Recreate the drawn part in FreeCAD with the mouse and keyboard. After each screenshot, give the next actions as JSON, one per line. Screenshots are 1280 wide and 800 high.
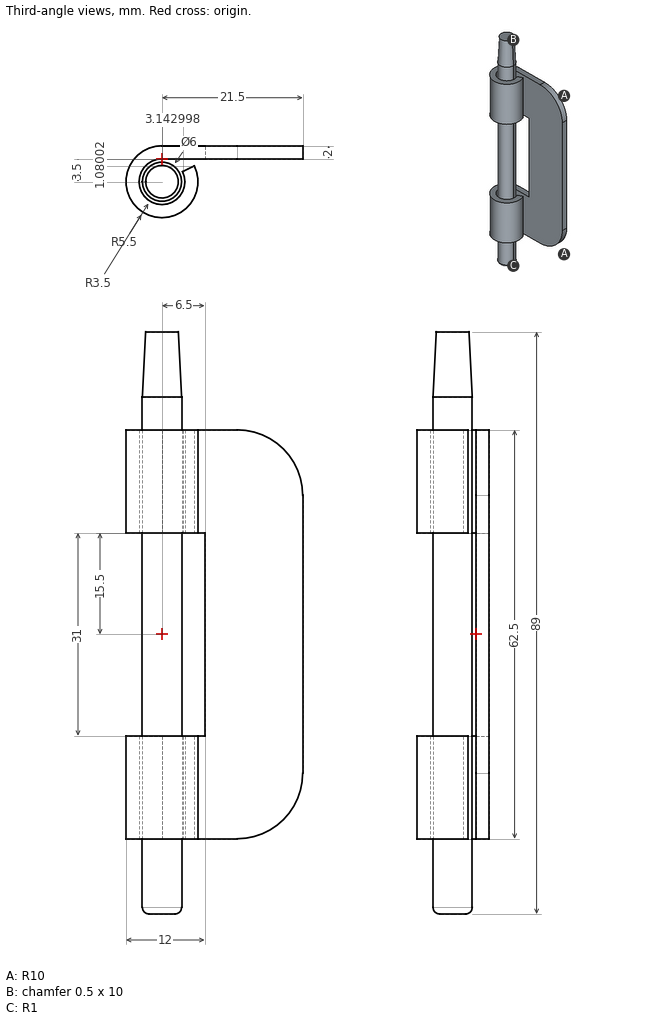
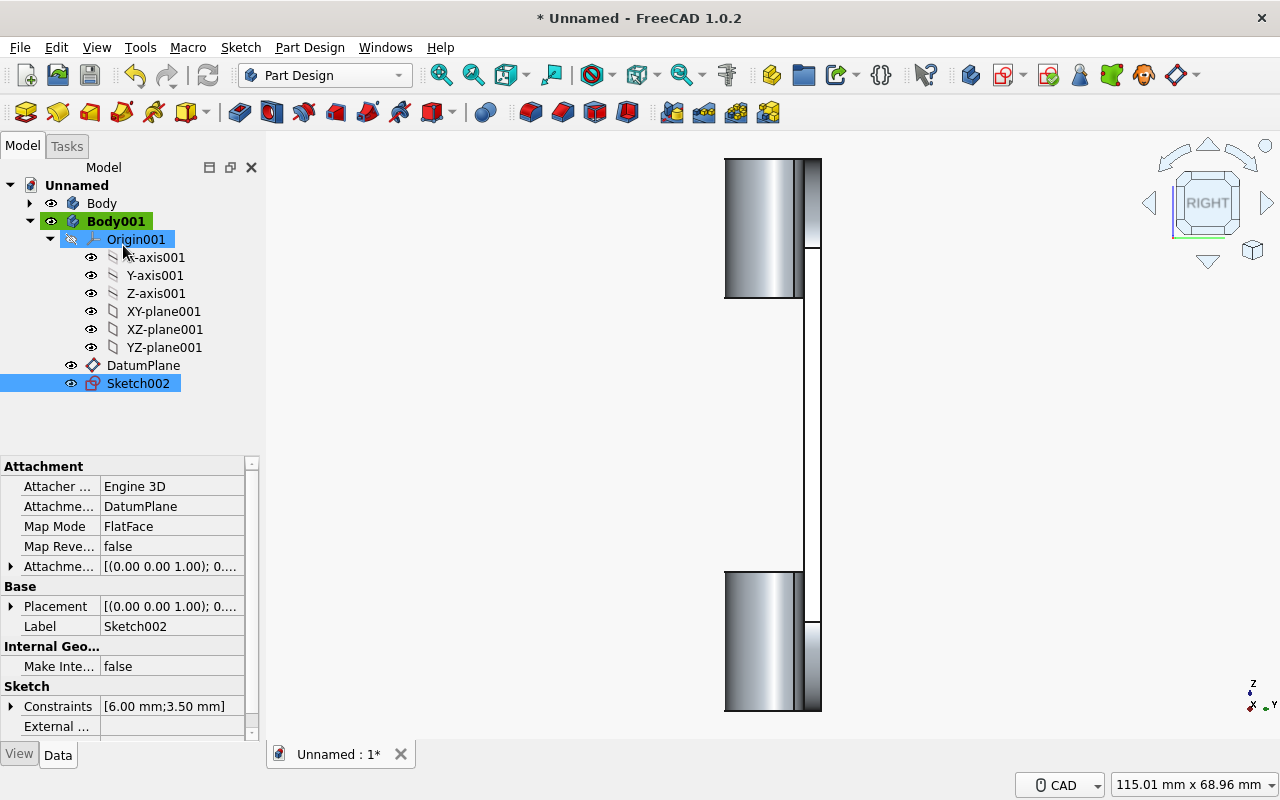
{"action": "left_click", "coordinate": [26, 112]}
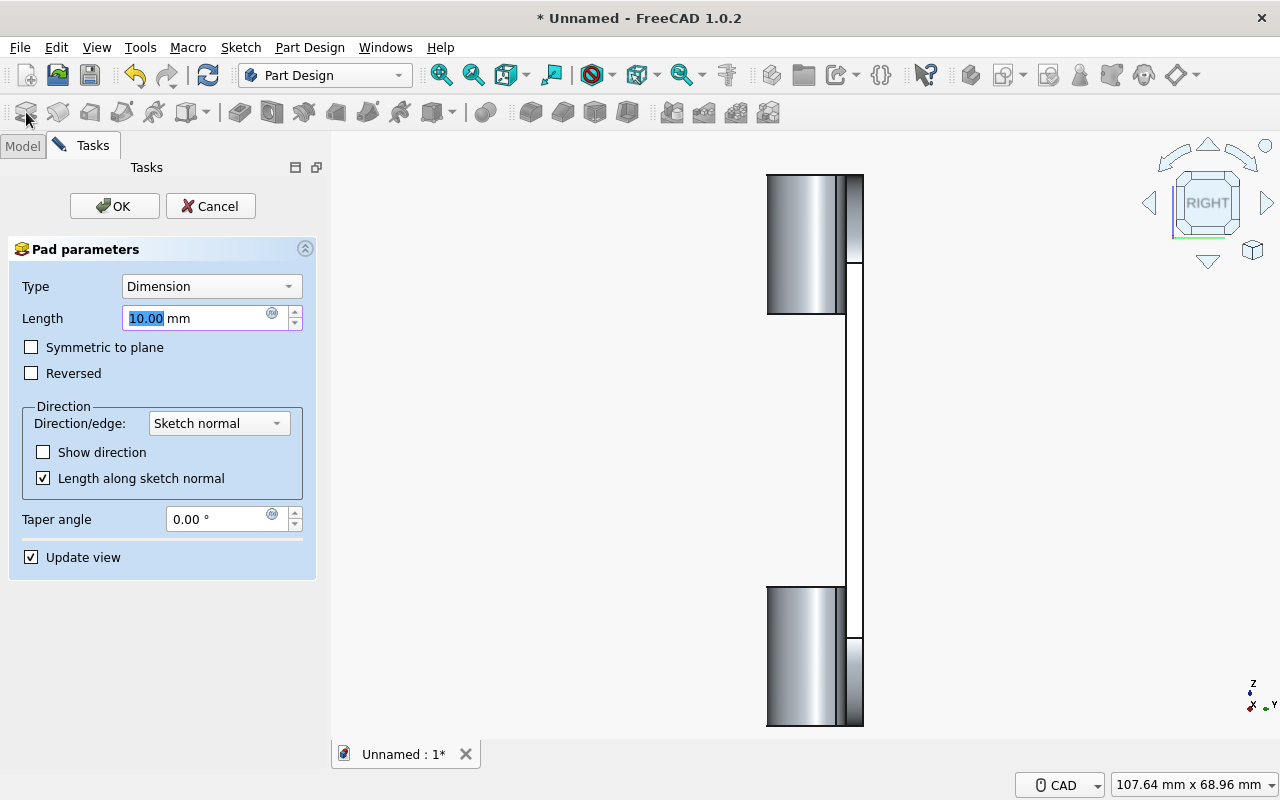
{"action": "type", "text": "89"}
{"action": "key", "text": "Tab"}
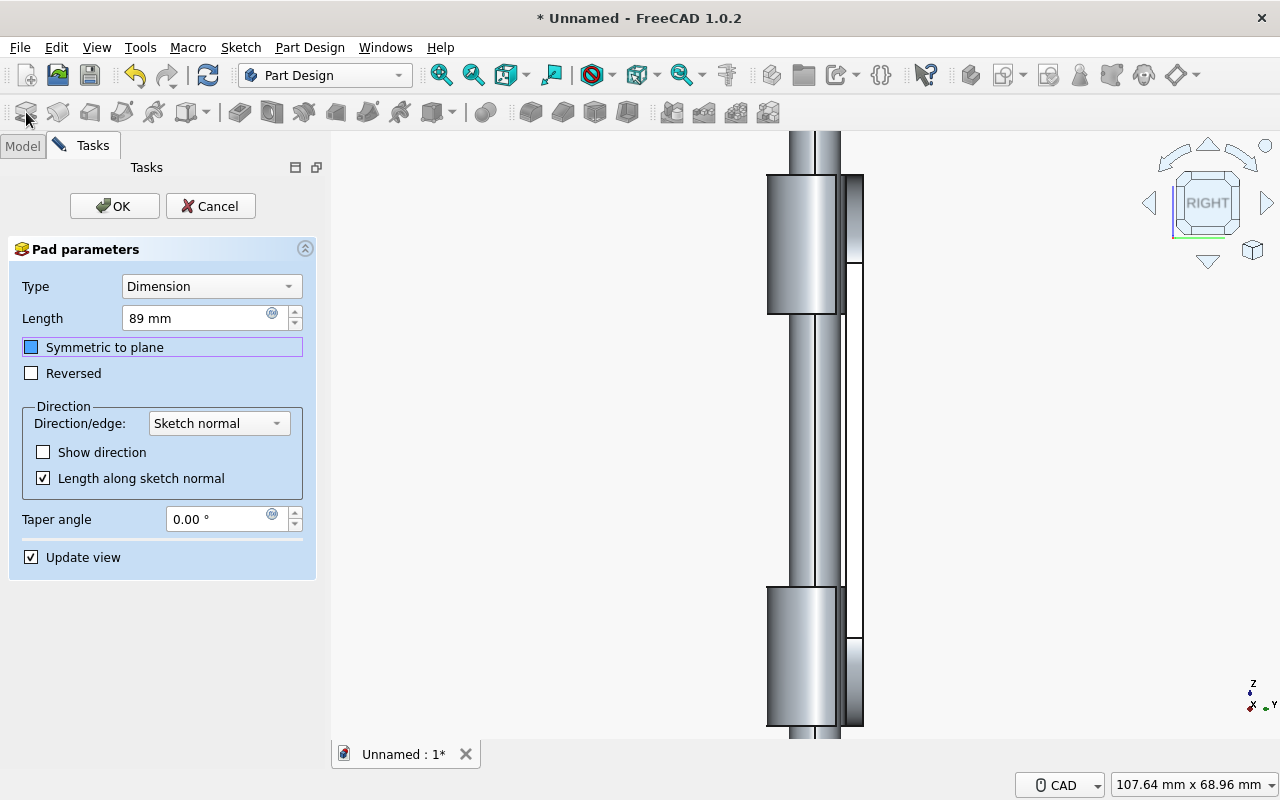
{"action": "left_click", "coordinate": [115, 206]}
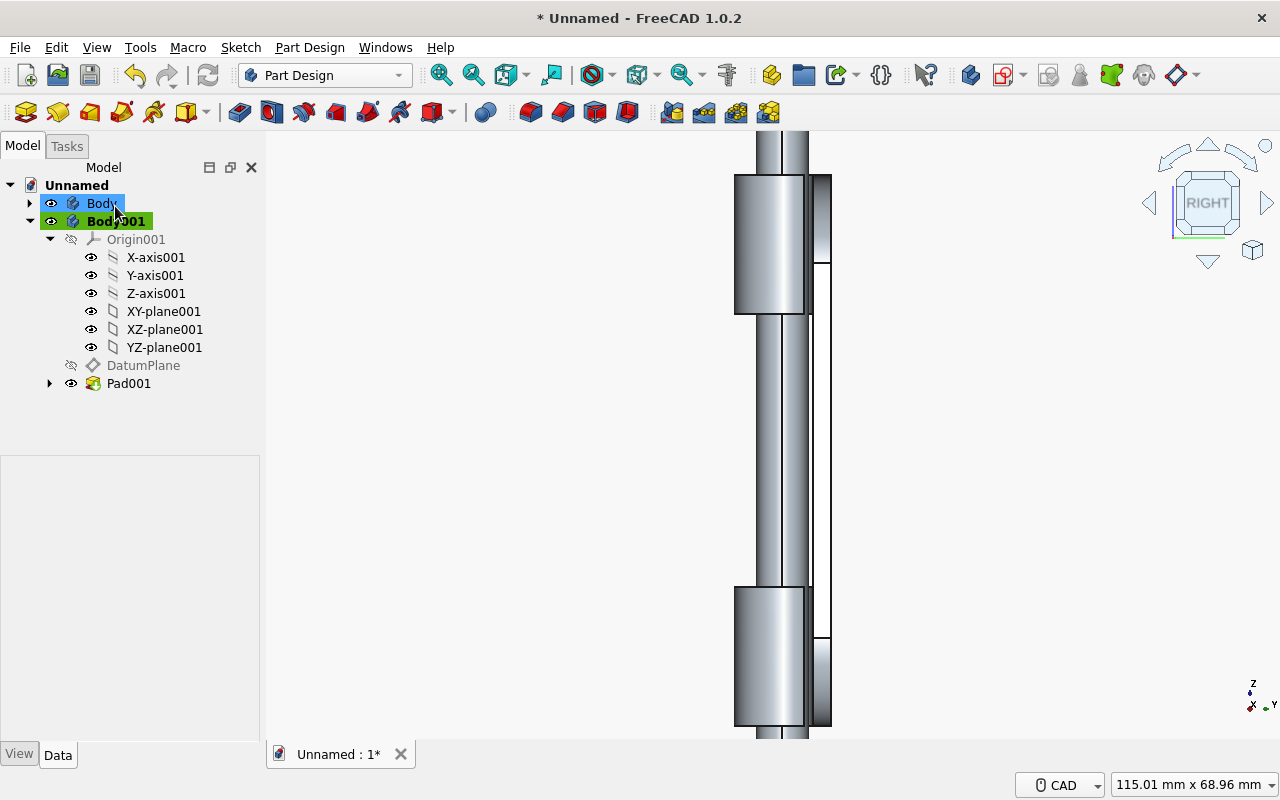
{"action": "key", "text": "v f"}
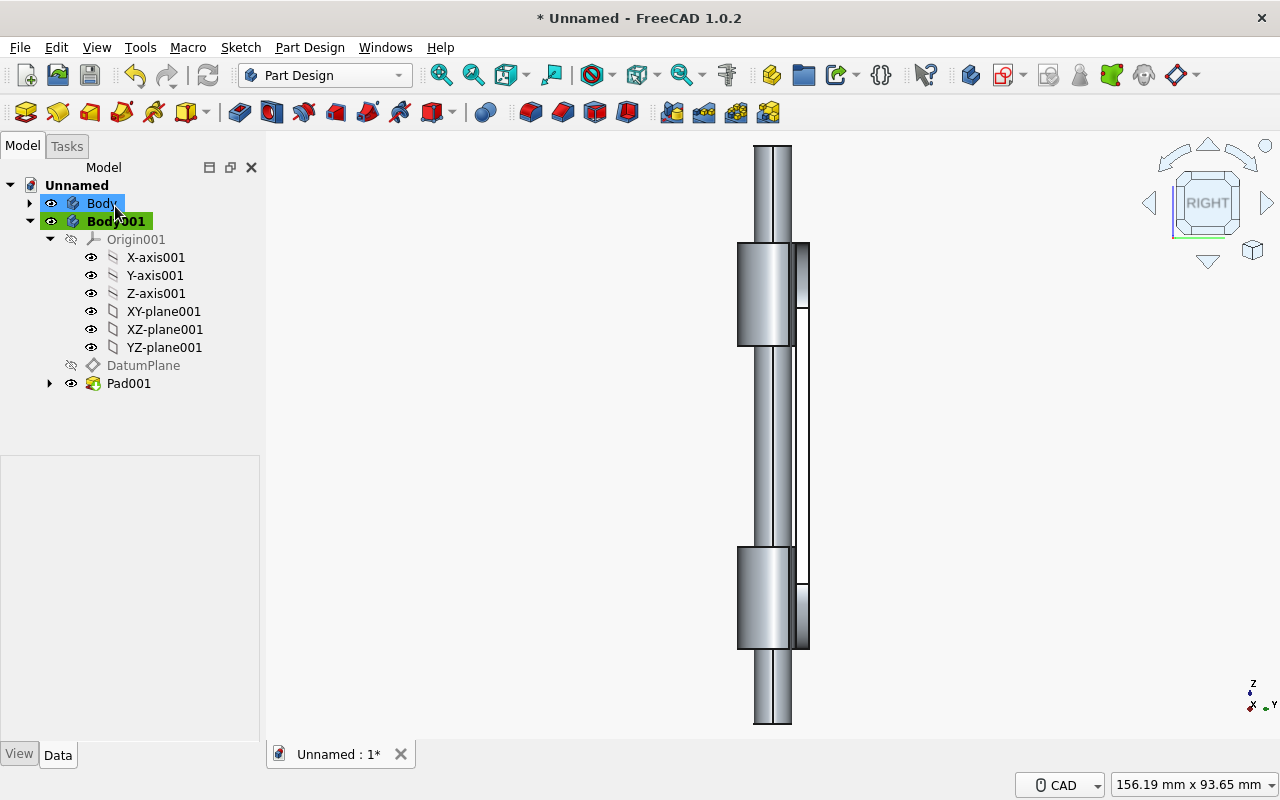
{"action": "key", "text": "0"}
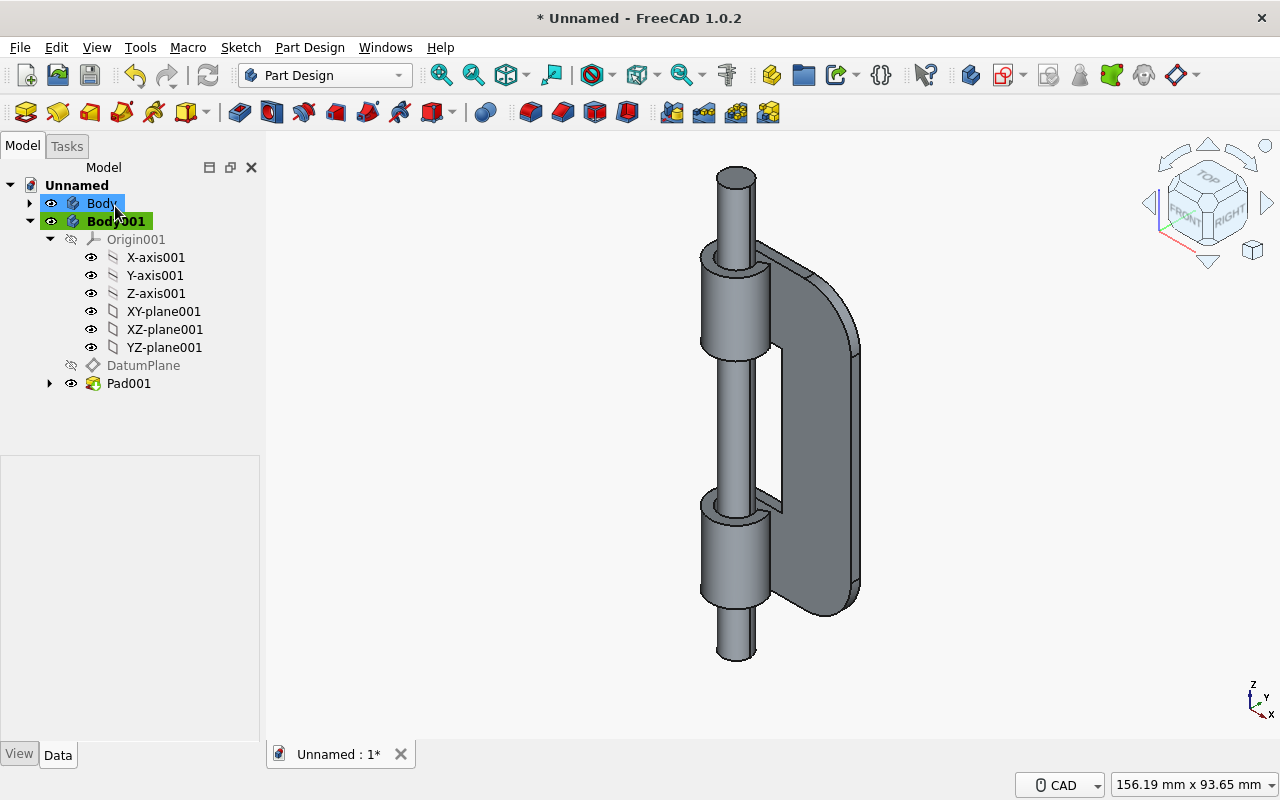
{"action": "left_click", "coordinate": [722, 169]}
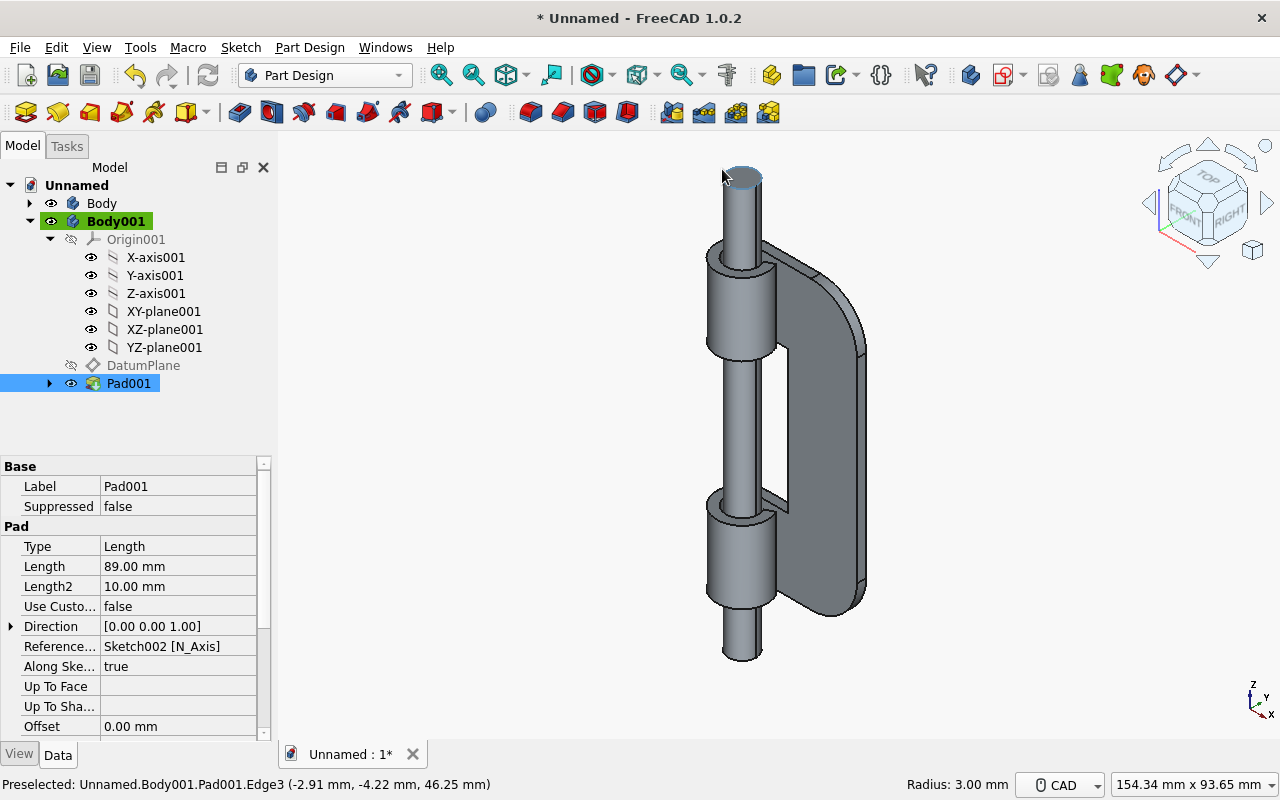
{"action": "left_click", "coordinate": [564, 112]}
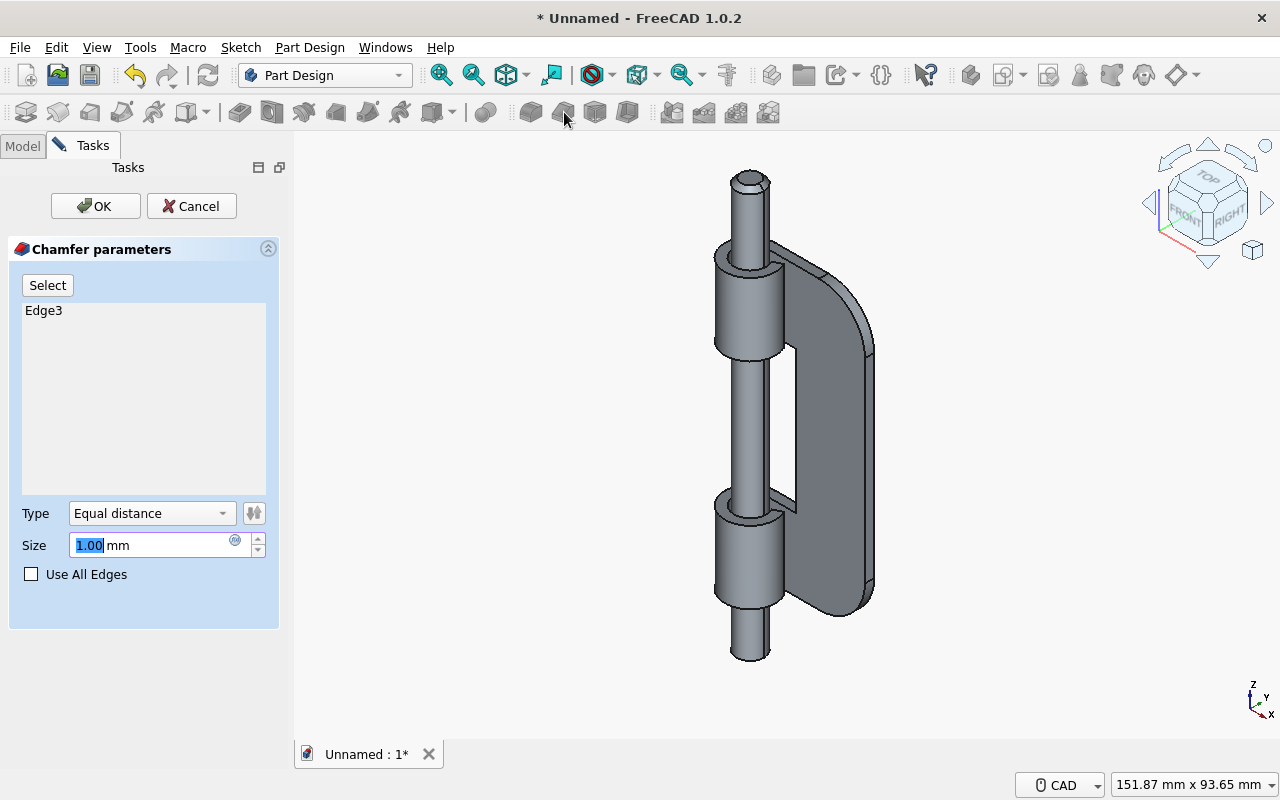
{"action": "type", "text": "0.5"}
{"action": "key", "text": "Tab"}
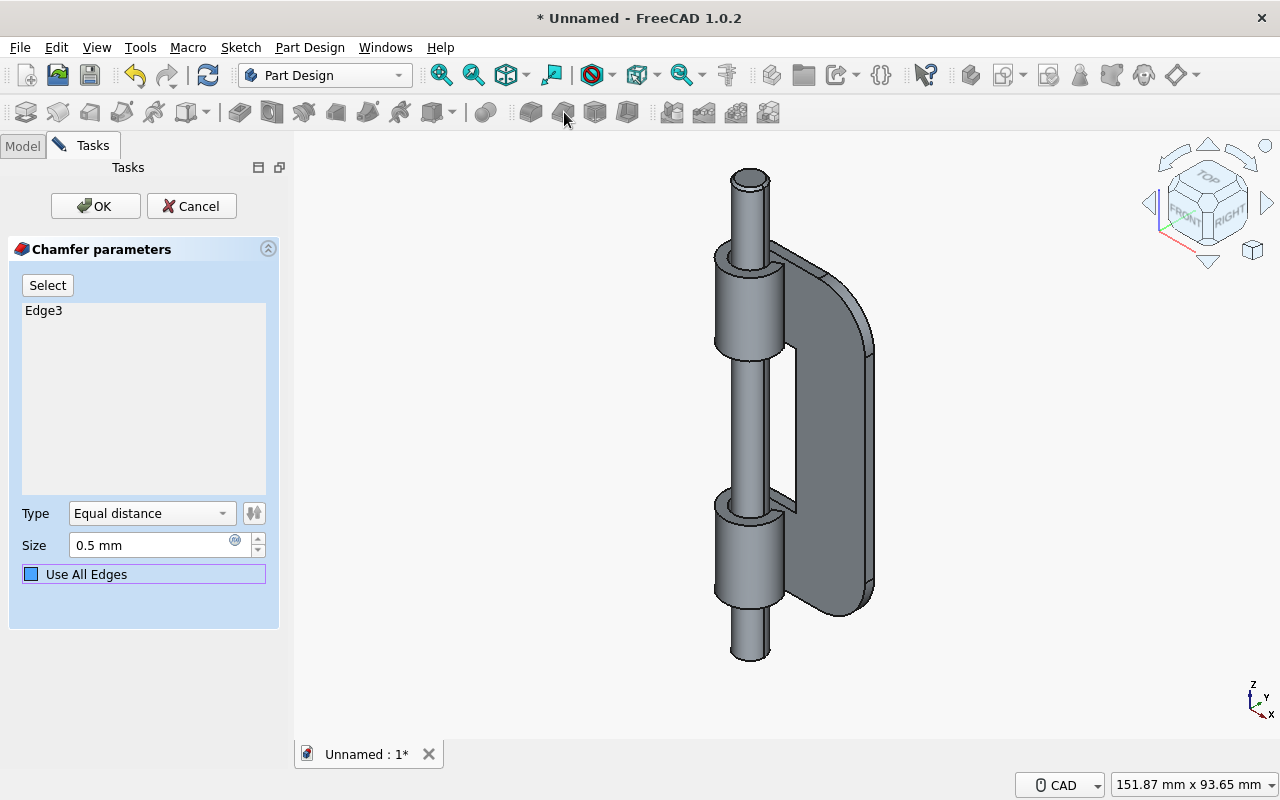
{"action": "left_click", "coordinate": [153, 514]}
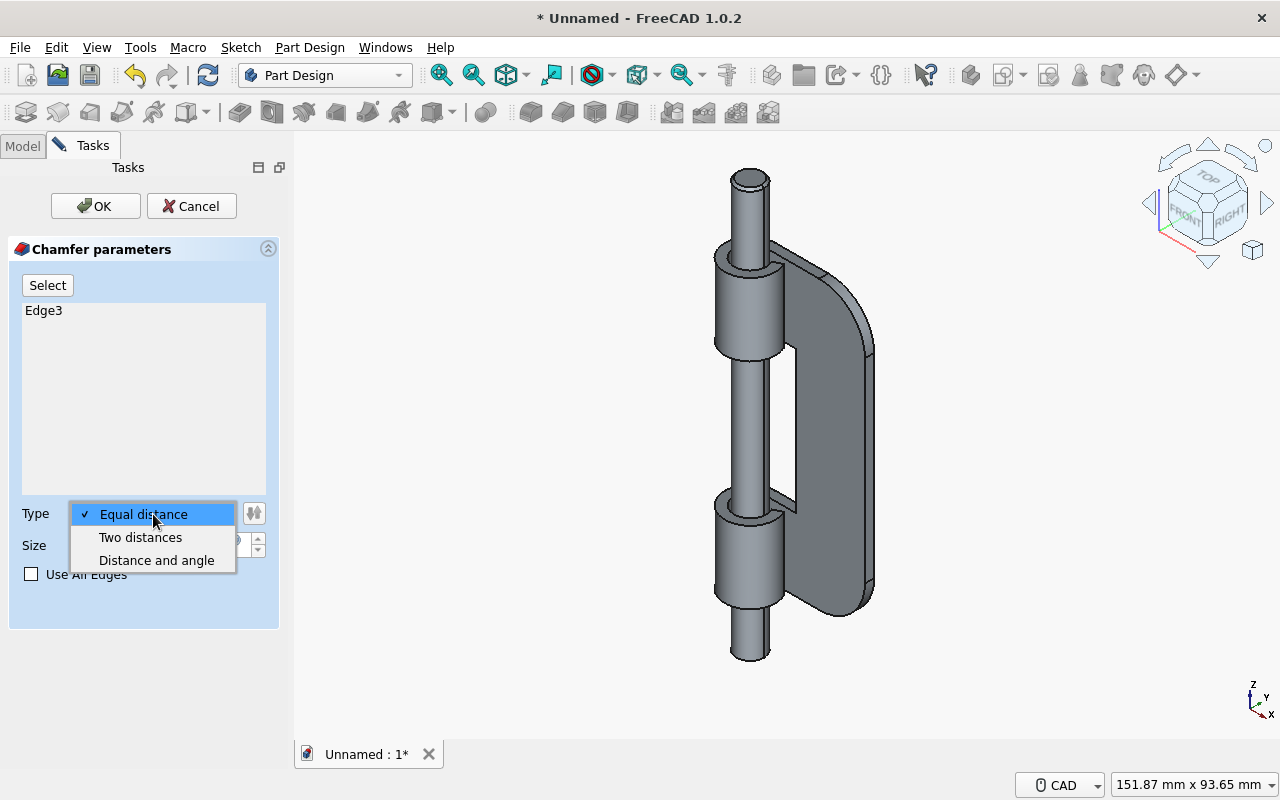
{"action": "left_click", "coordinate": [152, 538]}